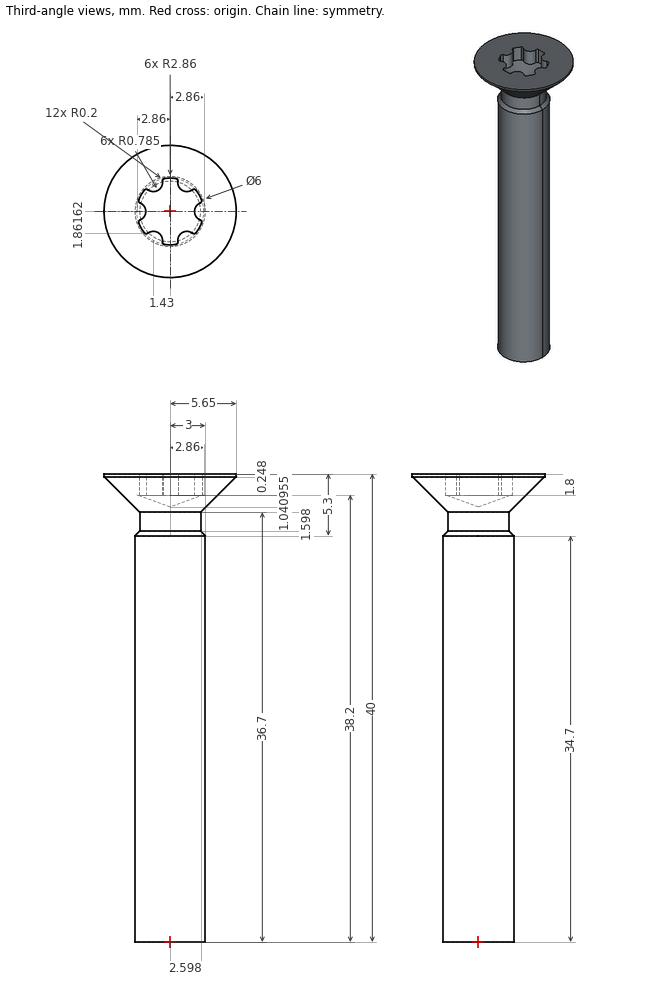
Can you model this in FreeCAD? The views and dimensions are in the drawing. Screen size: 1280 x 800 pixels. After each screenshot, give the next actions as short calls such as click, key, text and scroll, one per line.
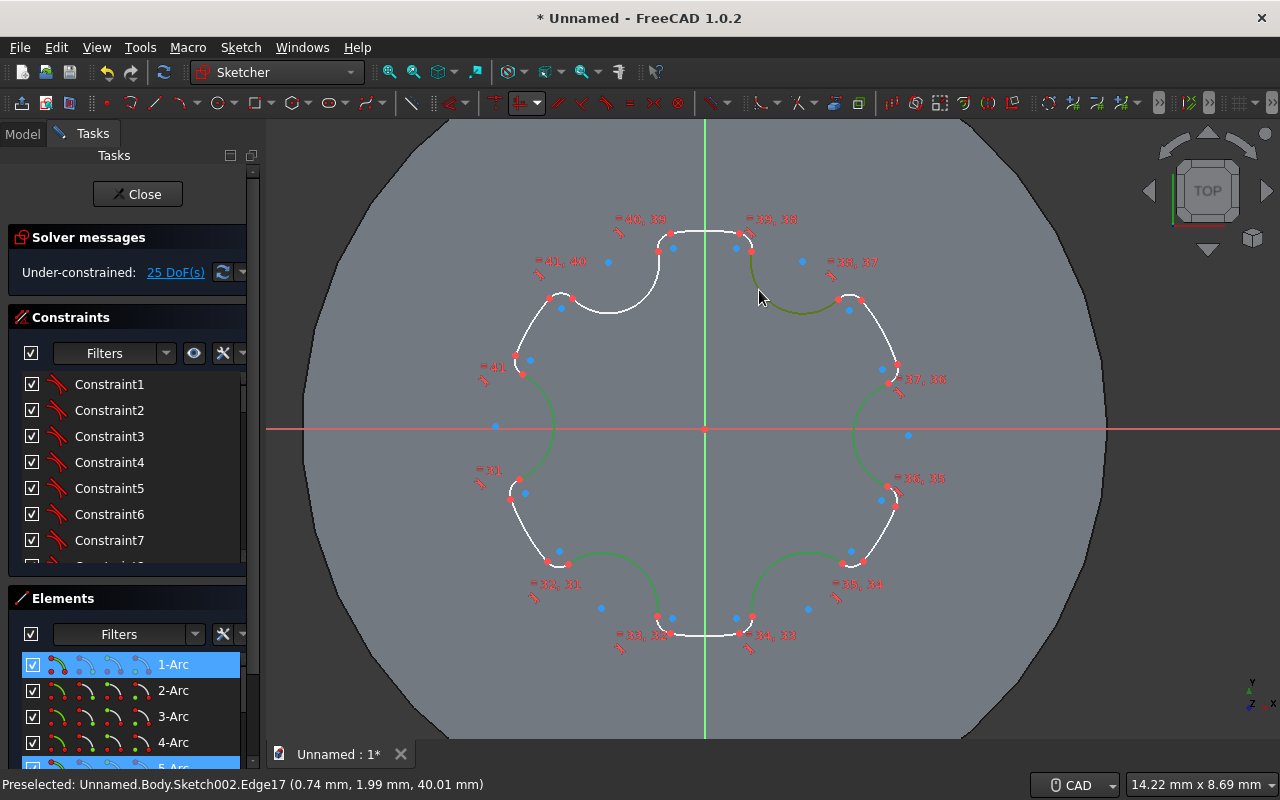
click(607, 313)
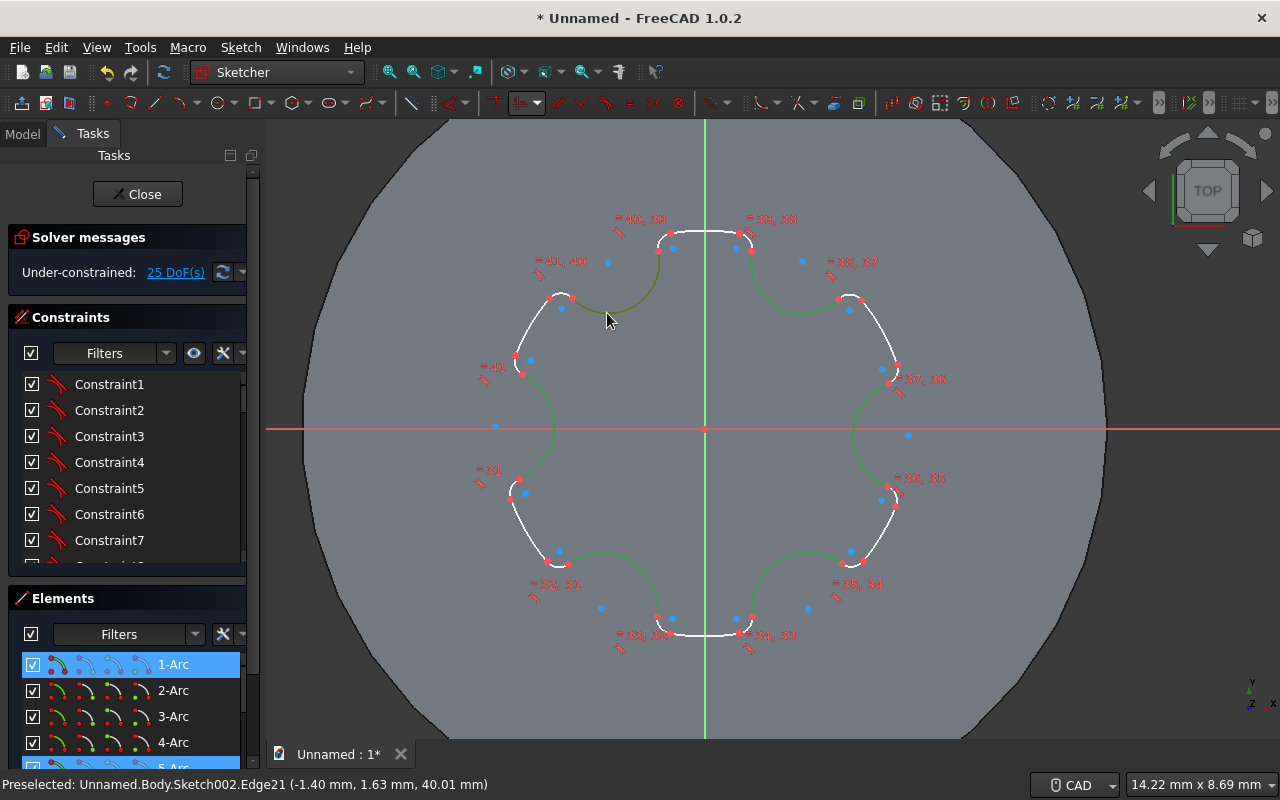
click(630, 104)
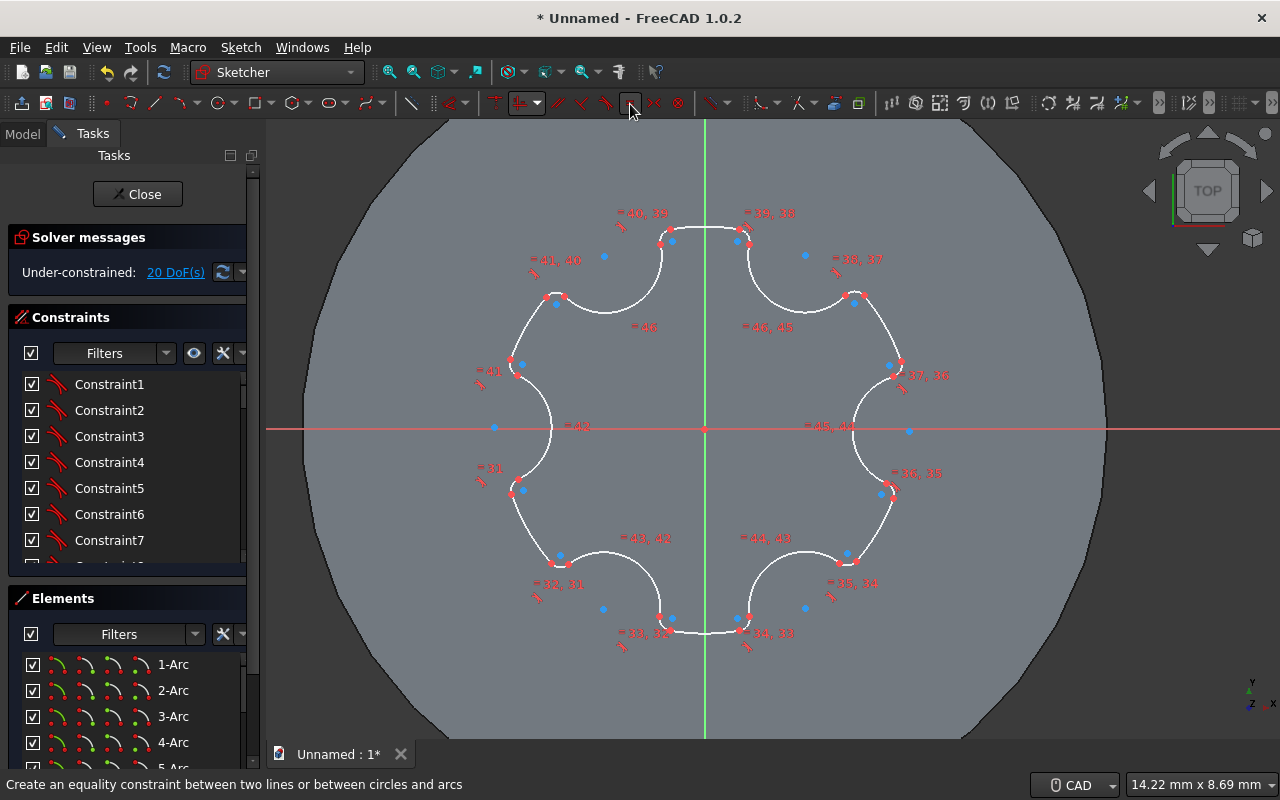
click(521, 516)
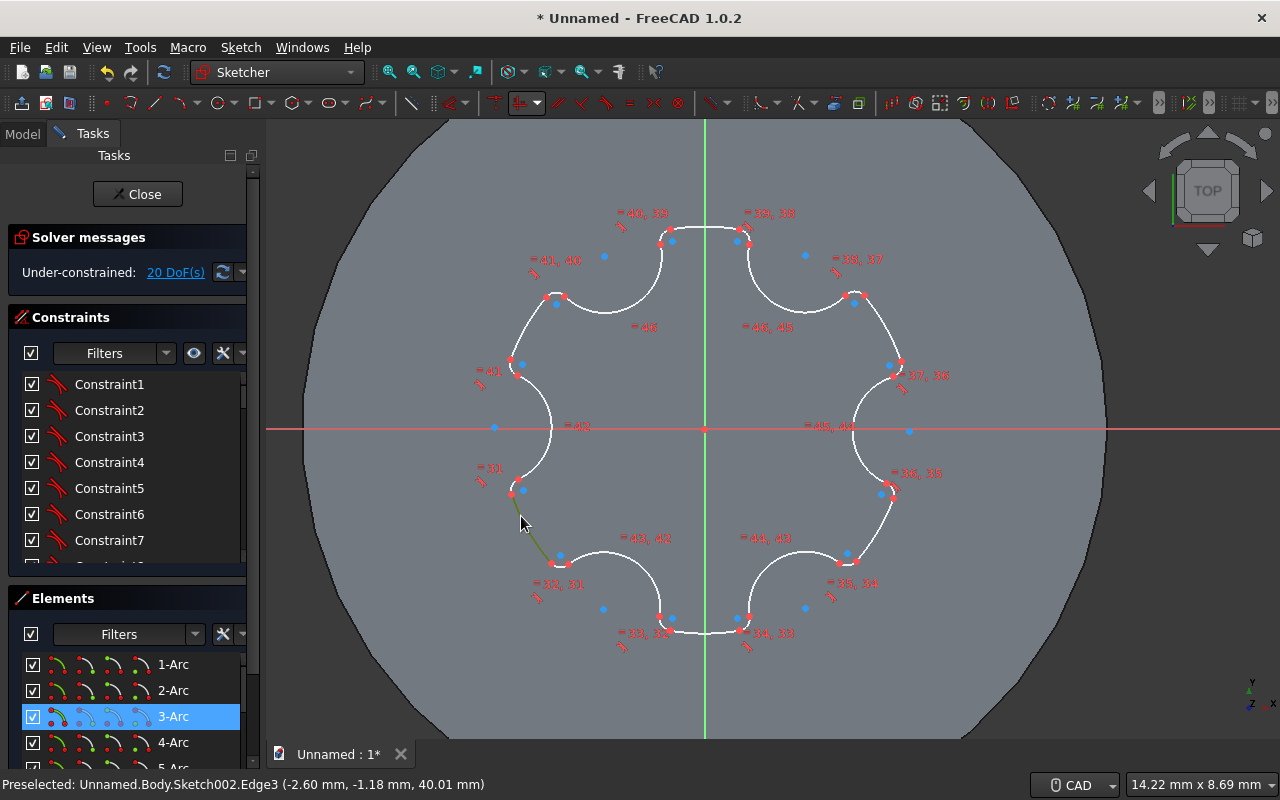
click(691, 633)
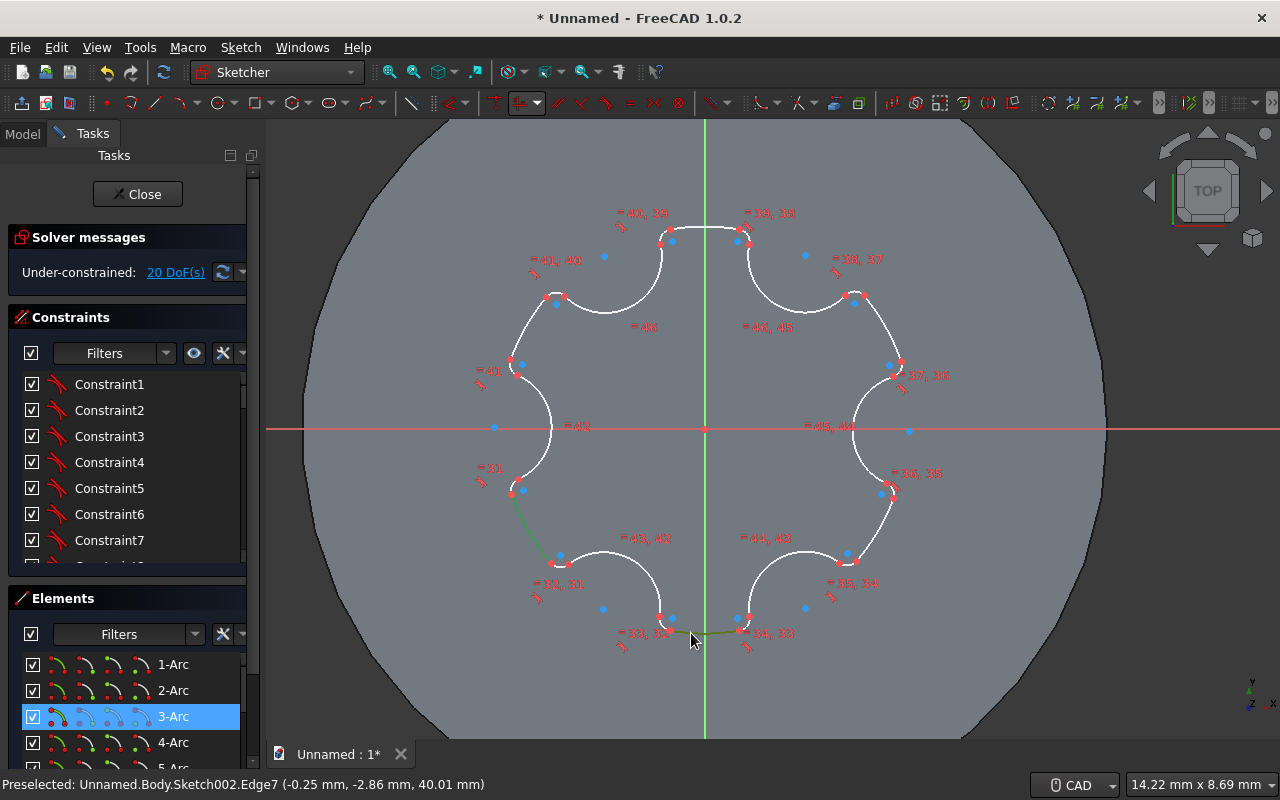
click(870, 544)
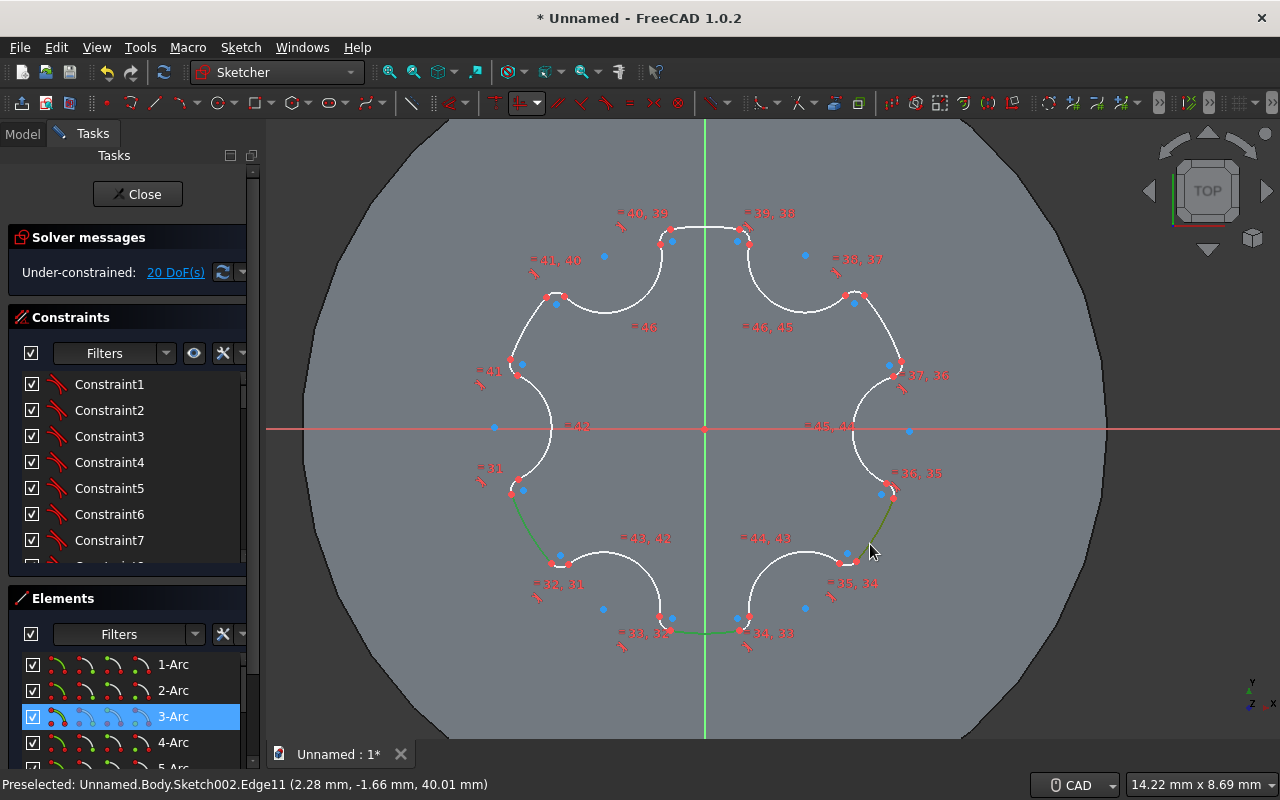
click(893, 340)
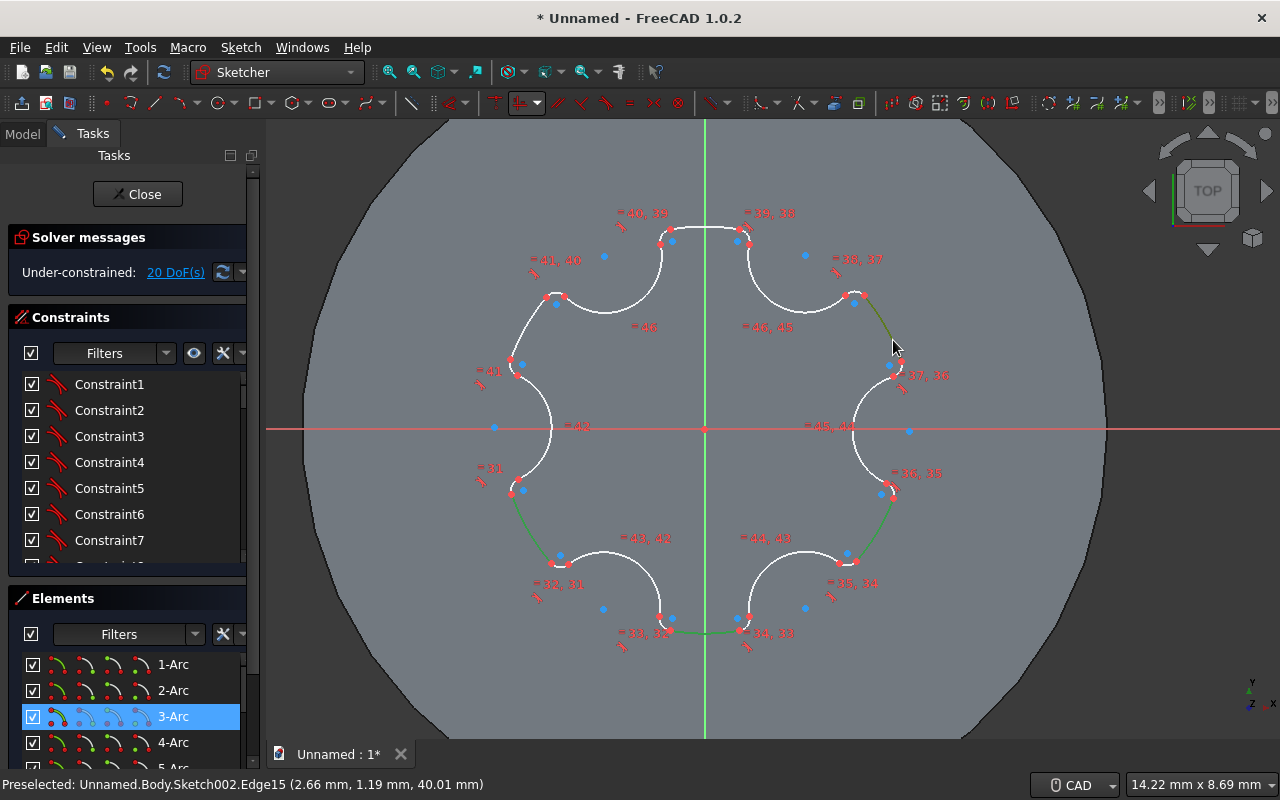
click(719, 227)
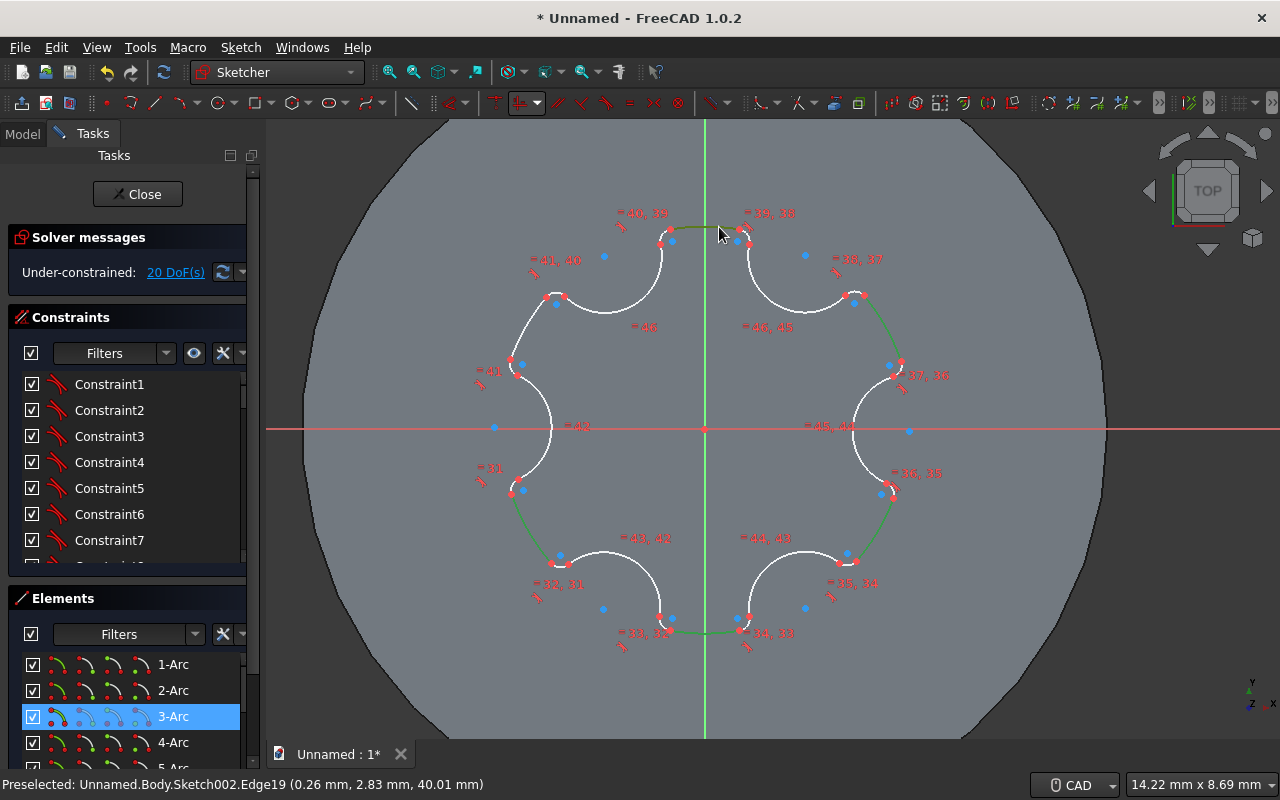
click(534, 314)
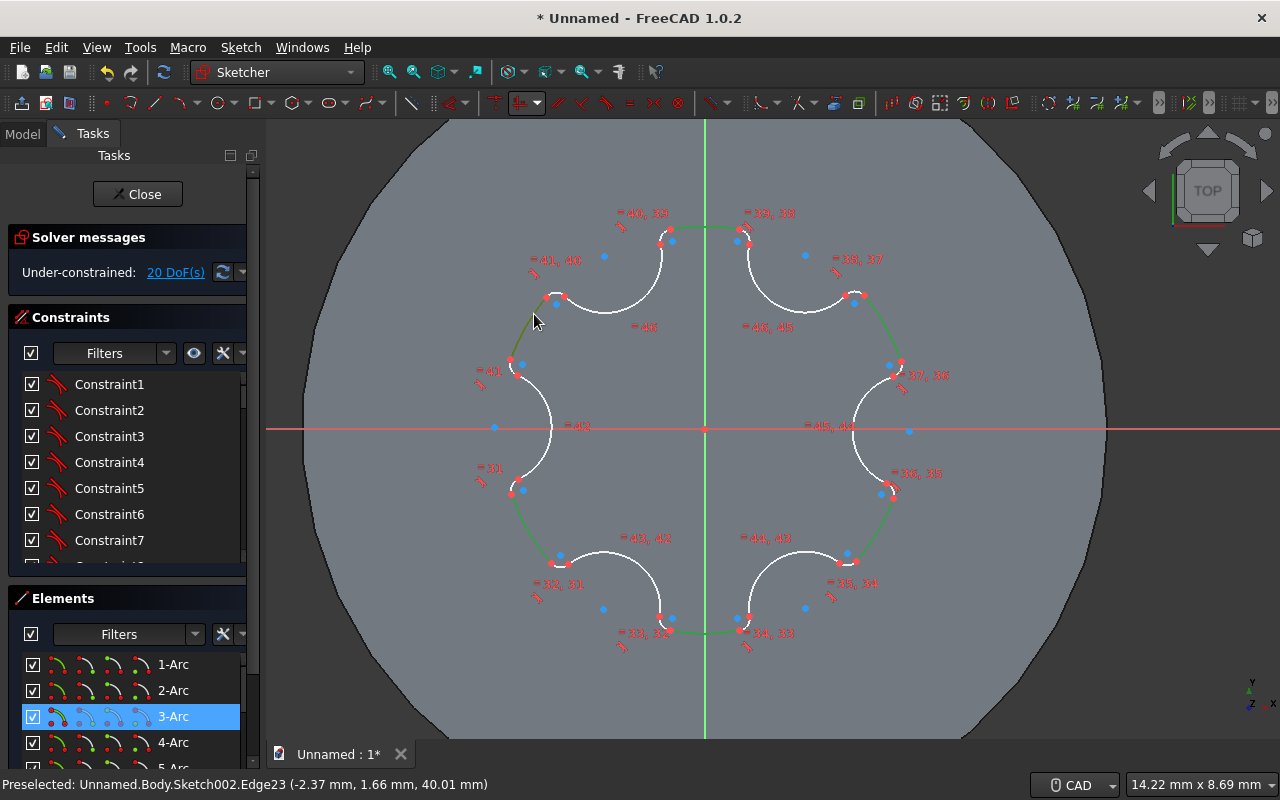
click(630, 104)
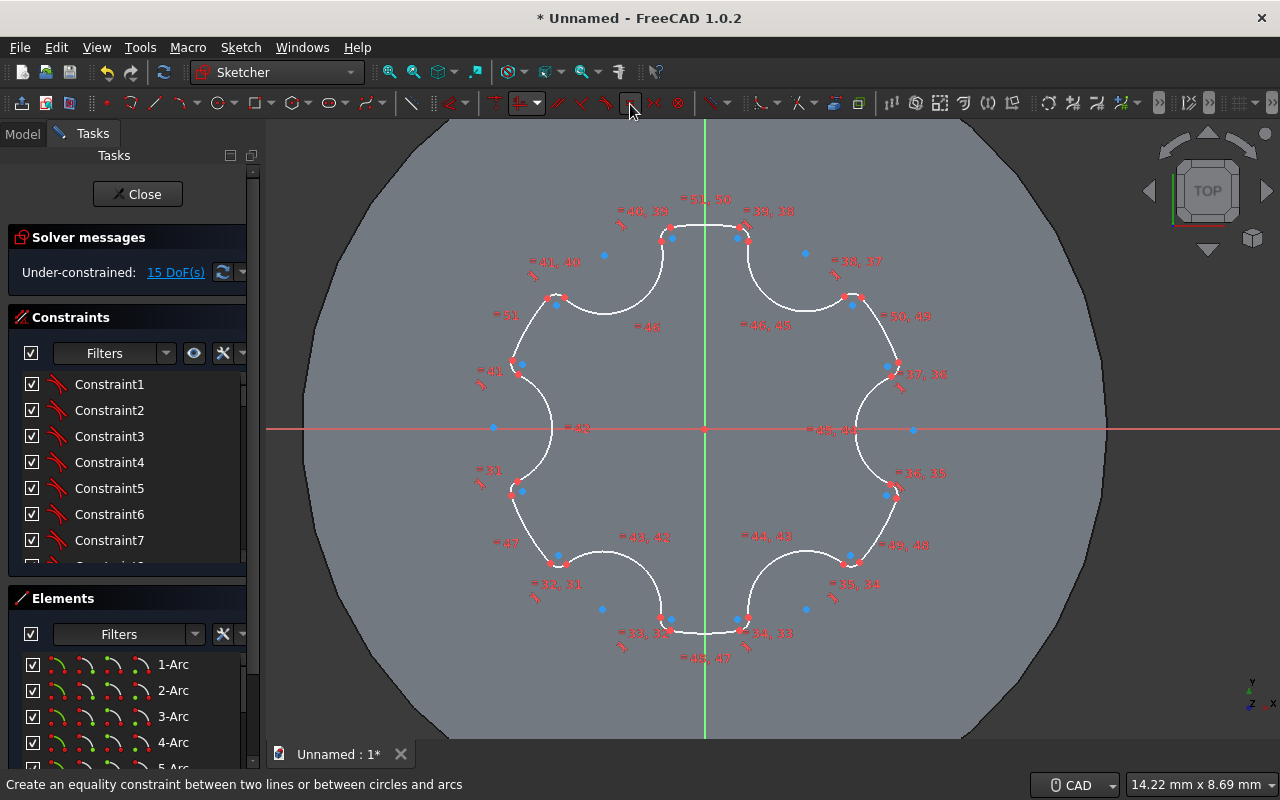
click(494, 428)